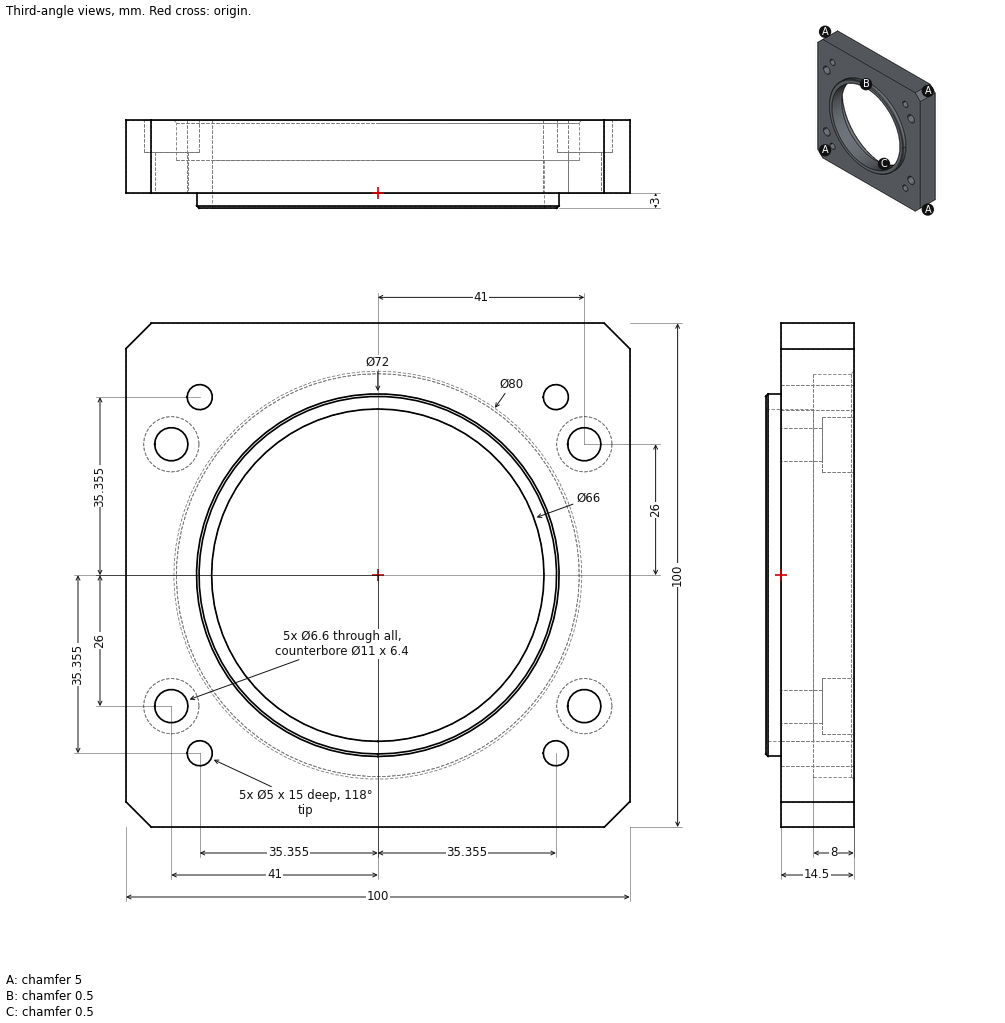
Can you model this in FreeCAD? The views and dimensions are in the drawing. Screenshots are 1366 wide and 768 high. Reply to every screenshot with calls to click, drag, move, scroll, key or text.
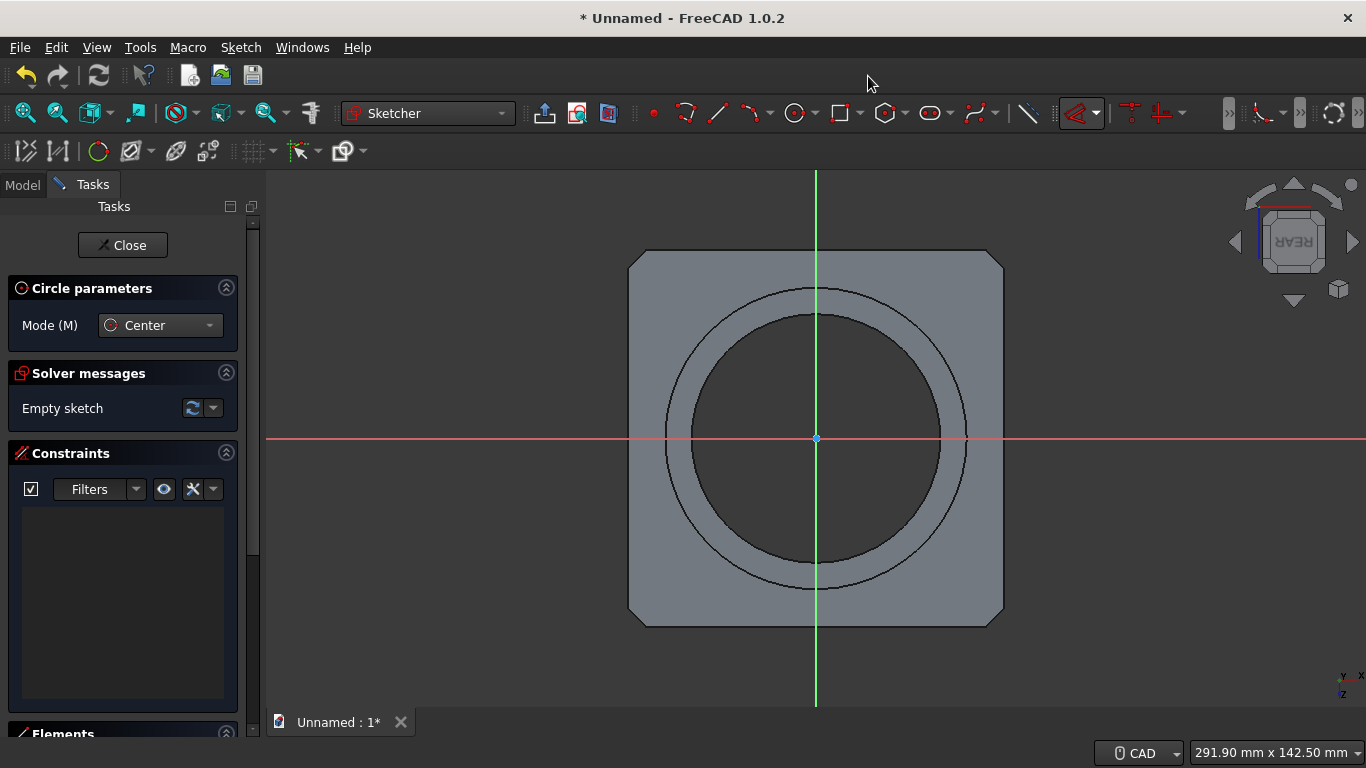
scroll(683, 305, up, 5)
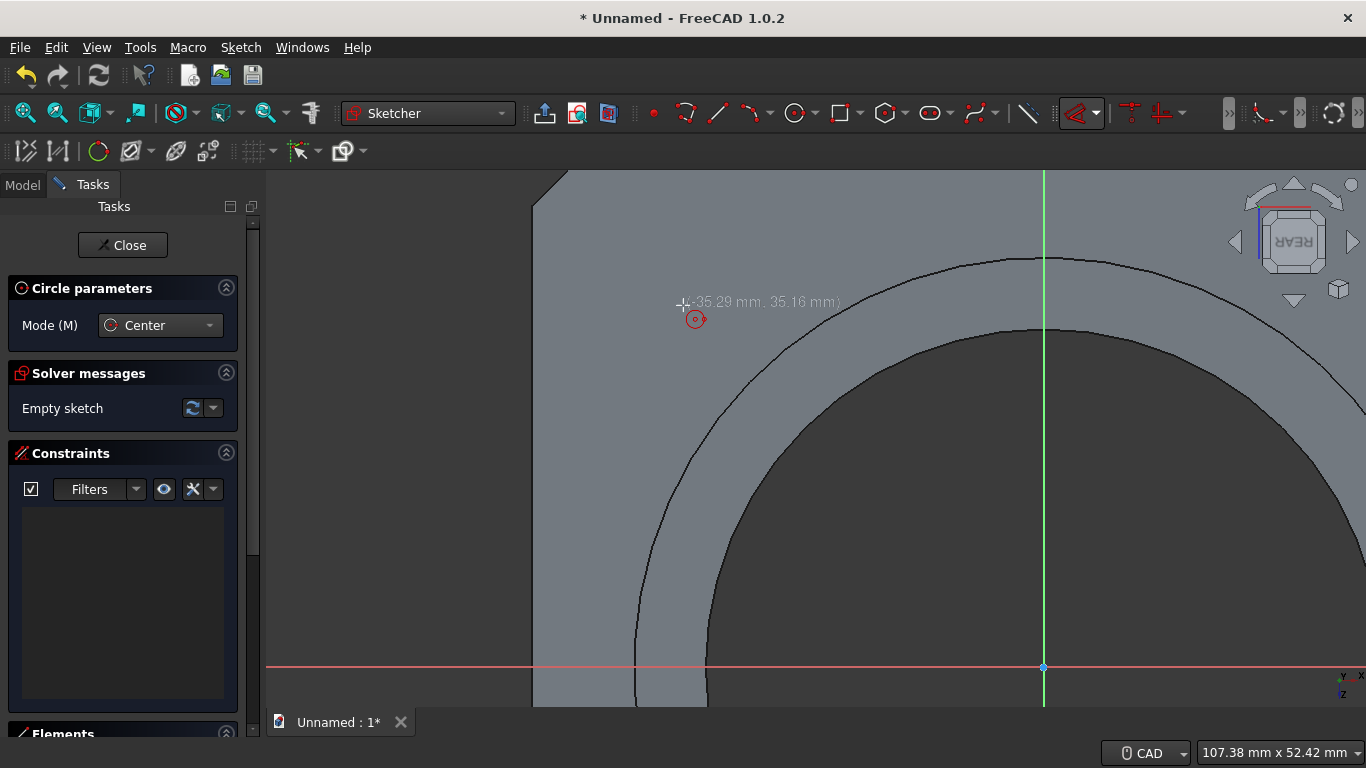
click(682, 305)
click(700, 287)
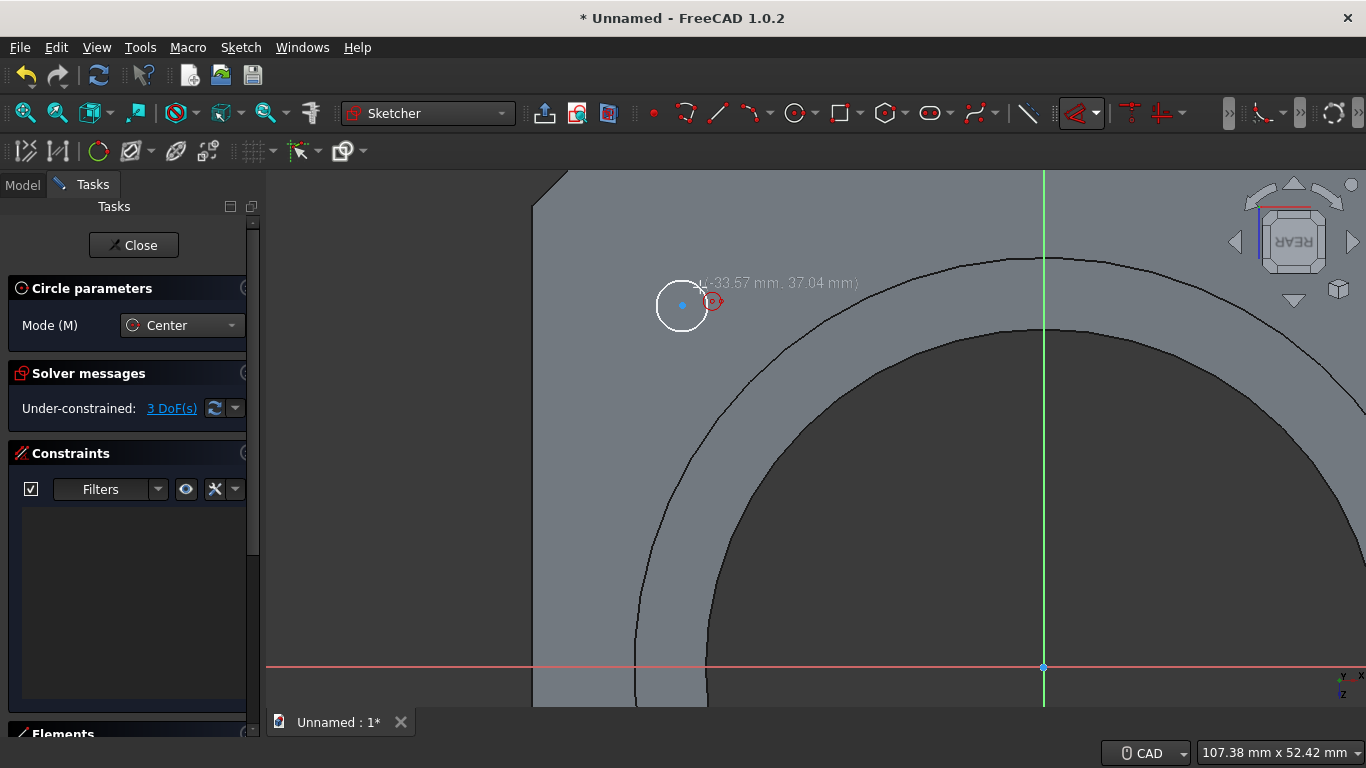
click(1044, 667)
click(1062, 649)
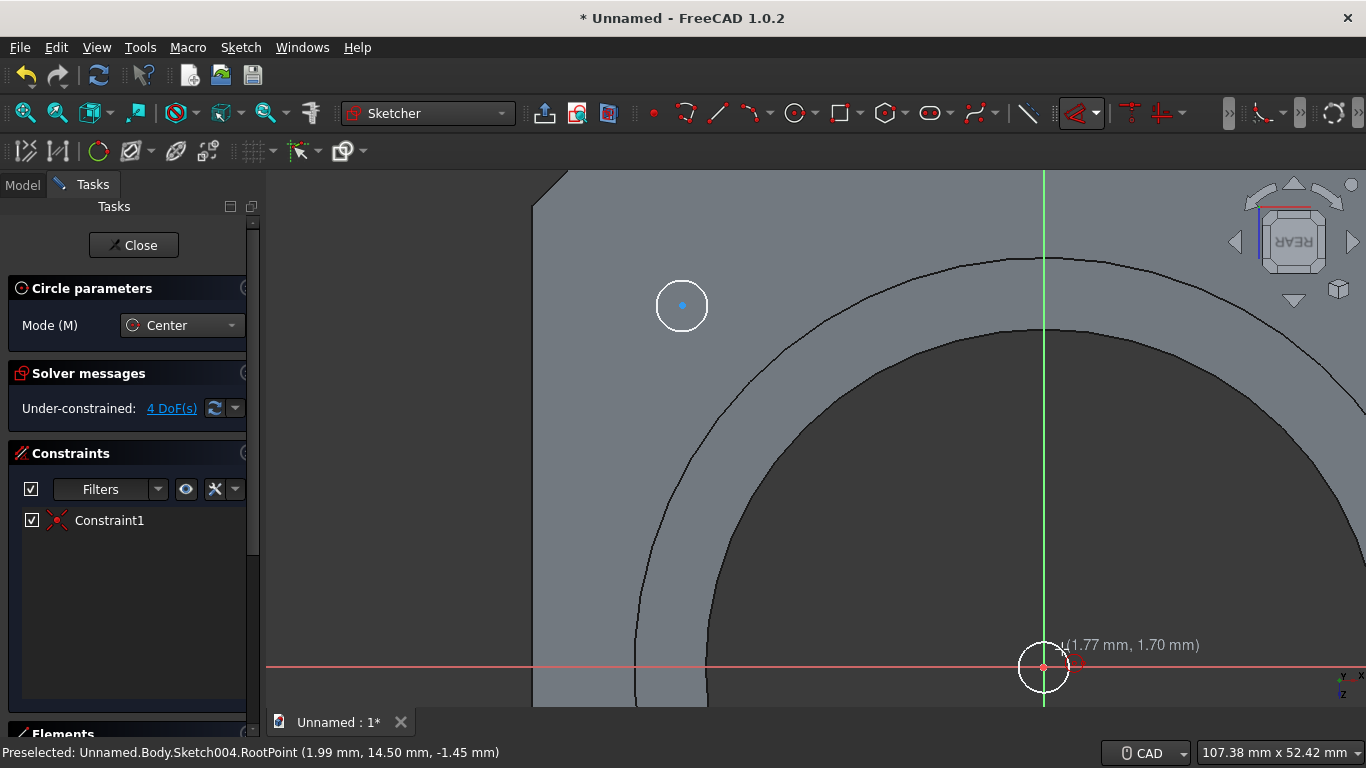
scroll(506, 252, down, 4)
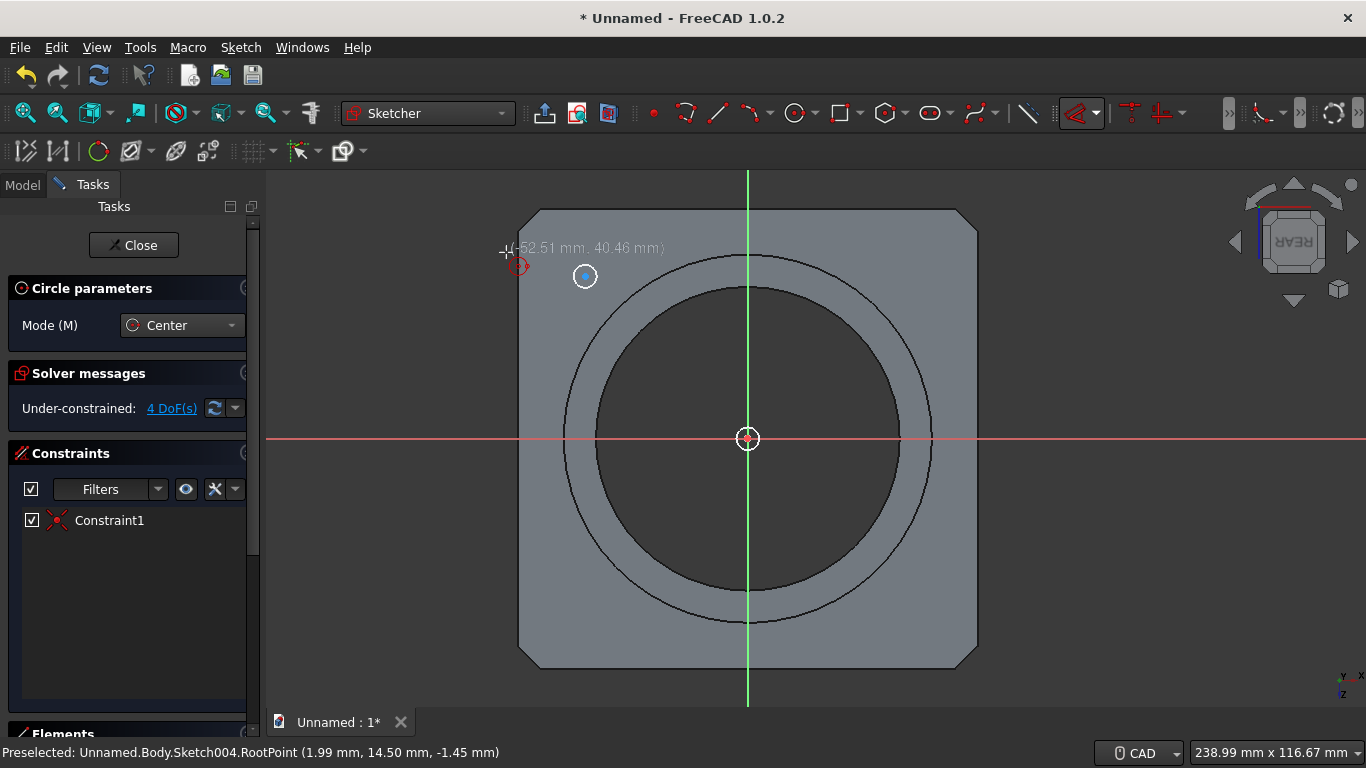
scroll(911, 276, up, 4)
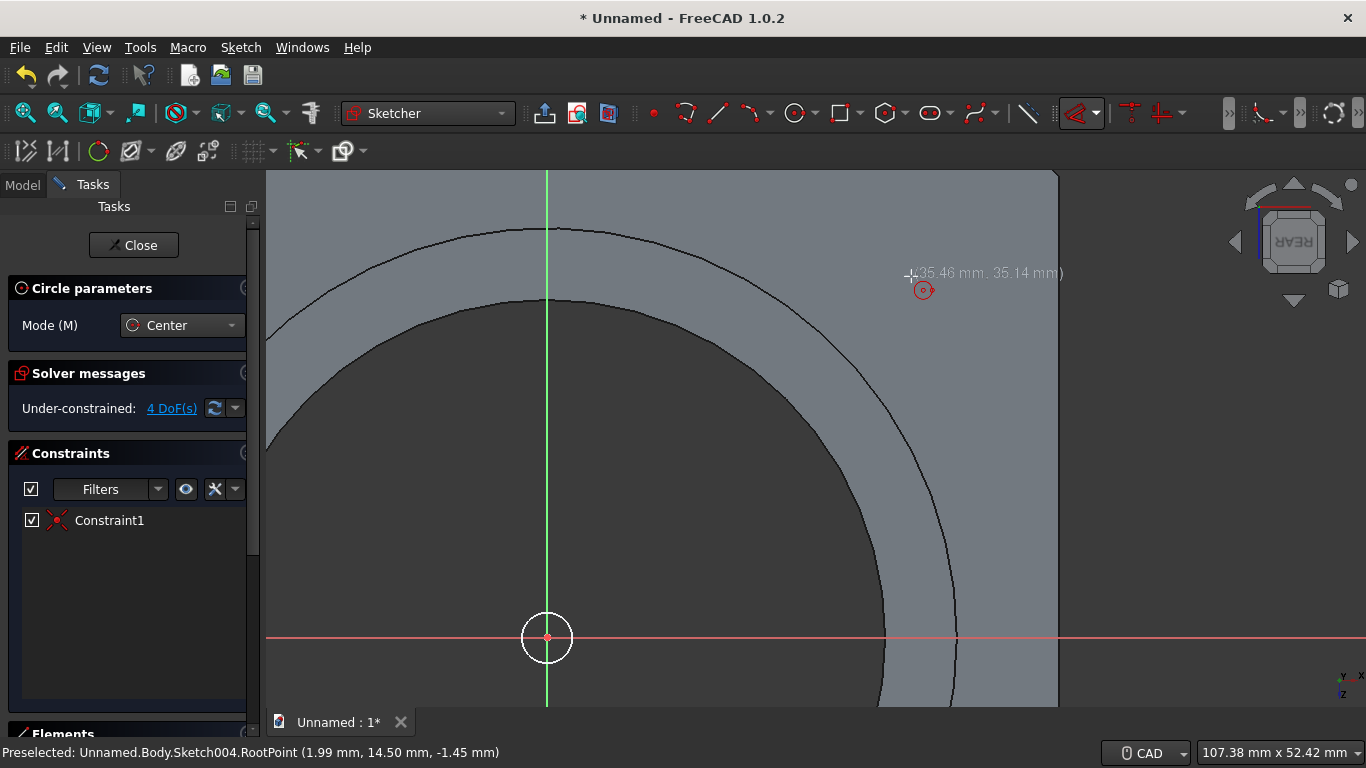
click(909, 276)
click(927, 258)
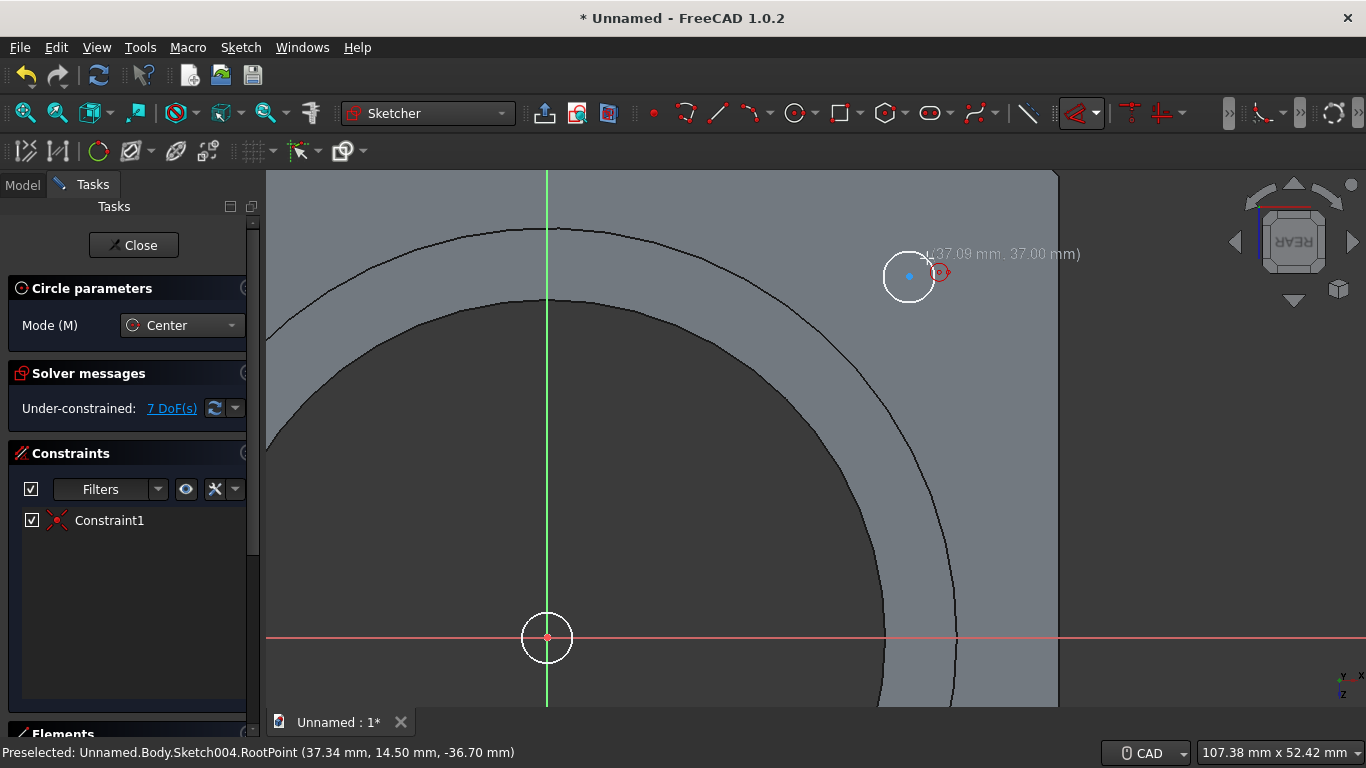
scroll(911, 276, down, 4)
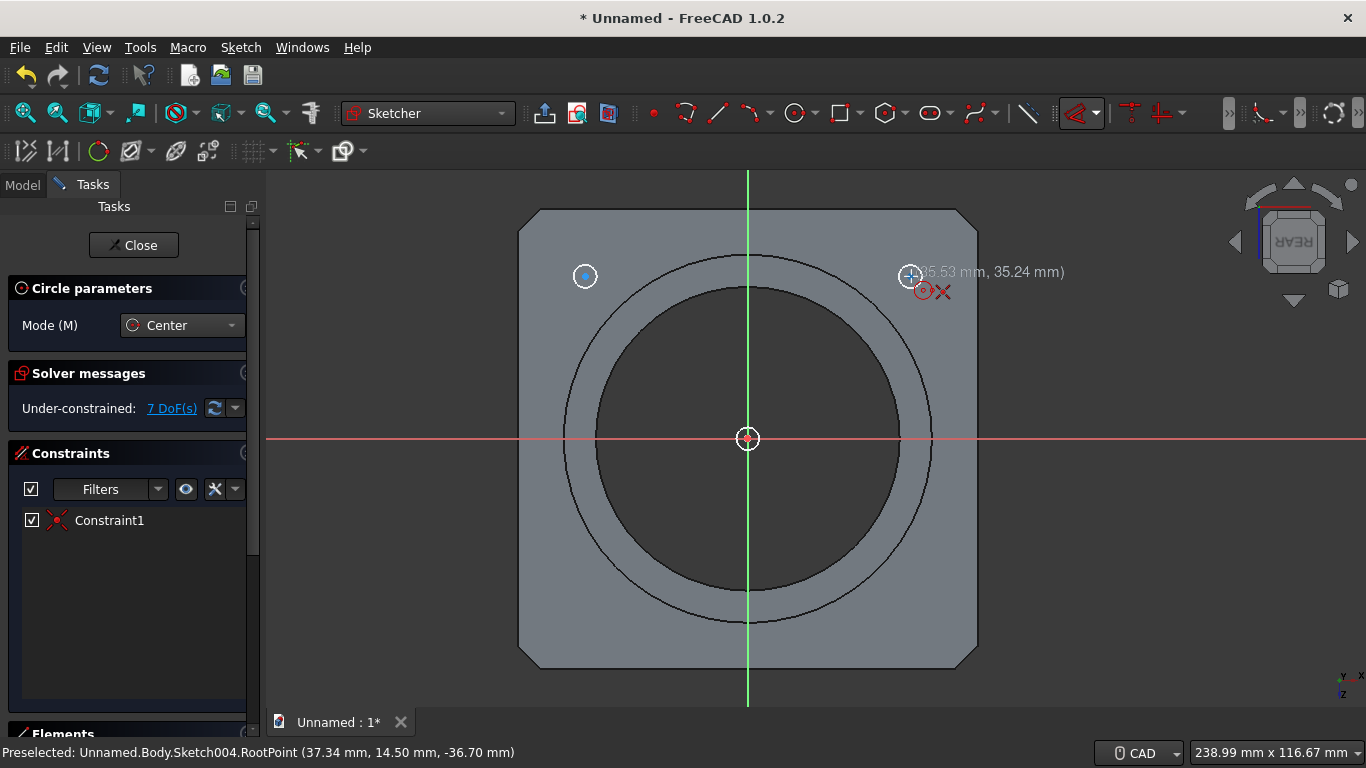
scroll(585, 601, up, 4)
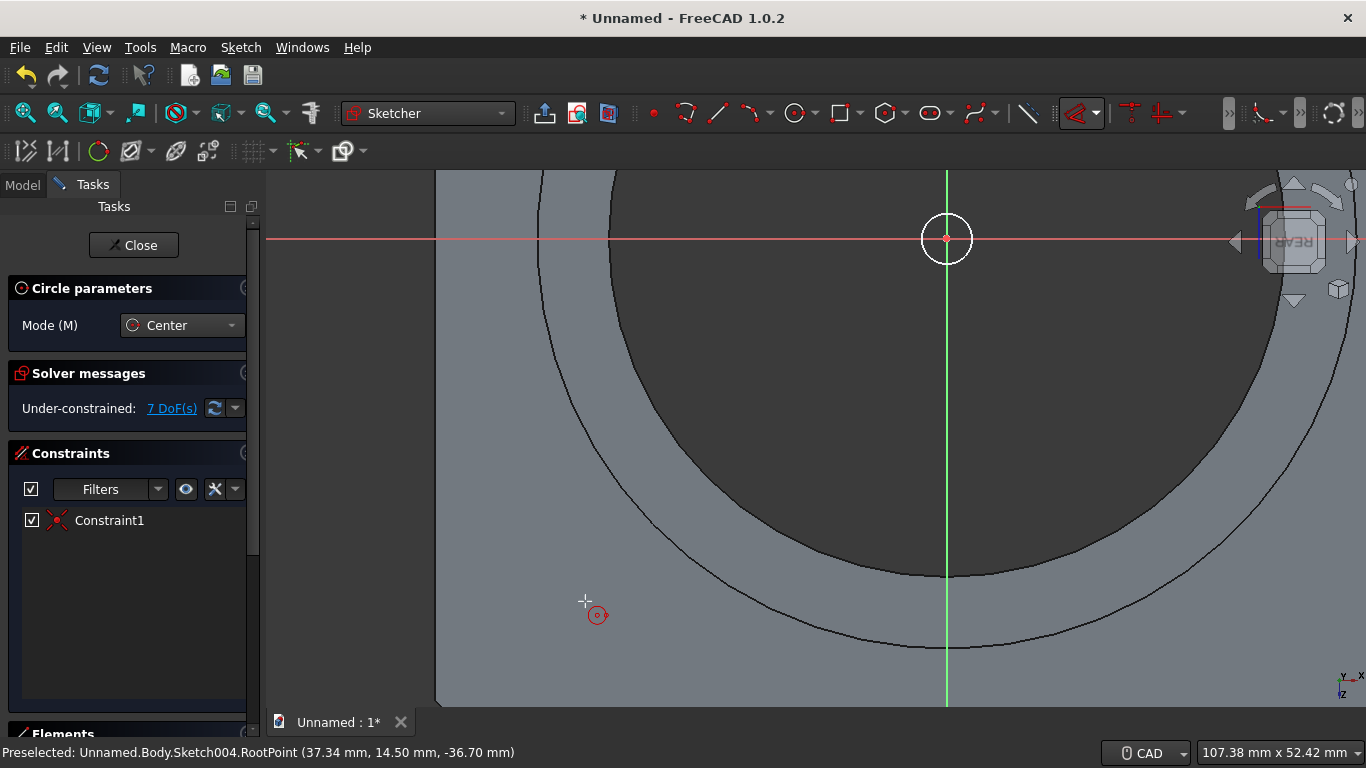
click(585, 601)
click(603, 583)